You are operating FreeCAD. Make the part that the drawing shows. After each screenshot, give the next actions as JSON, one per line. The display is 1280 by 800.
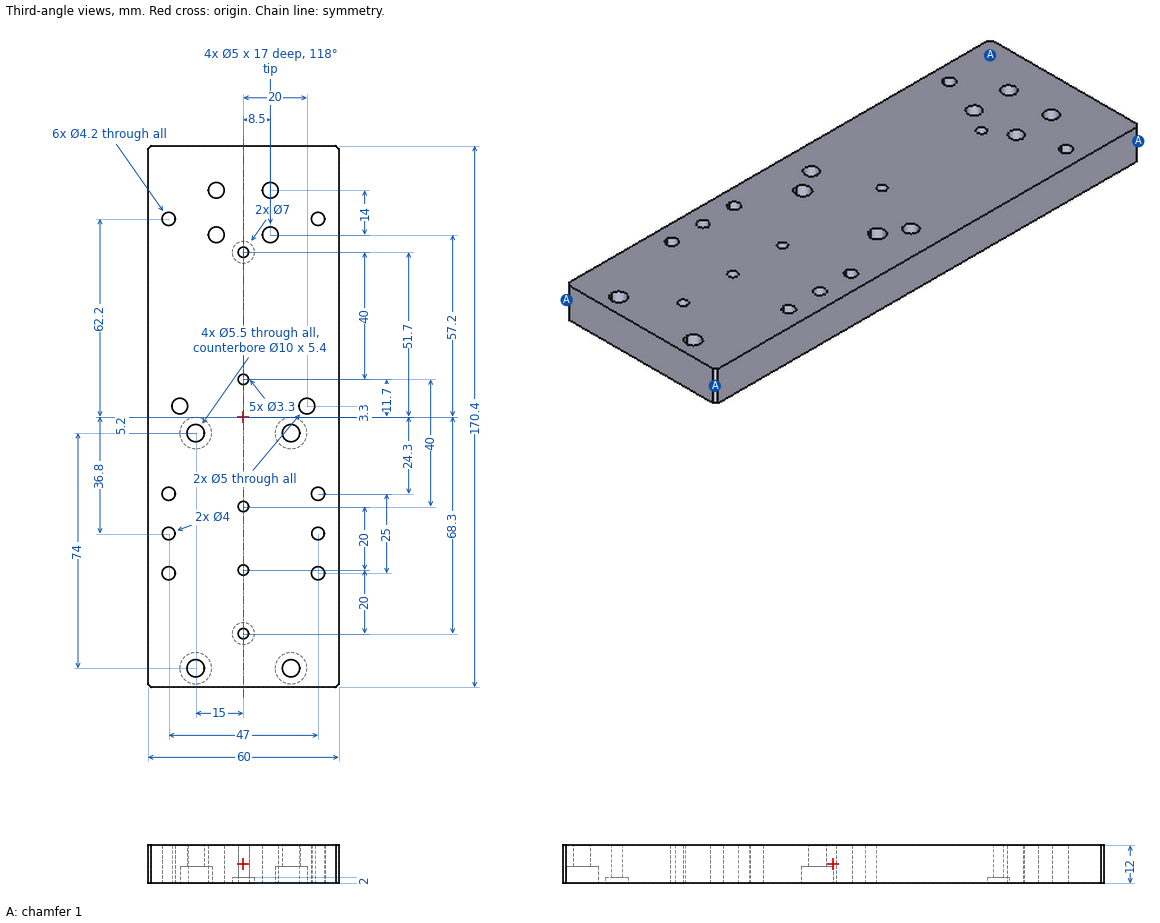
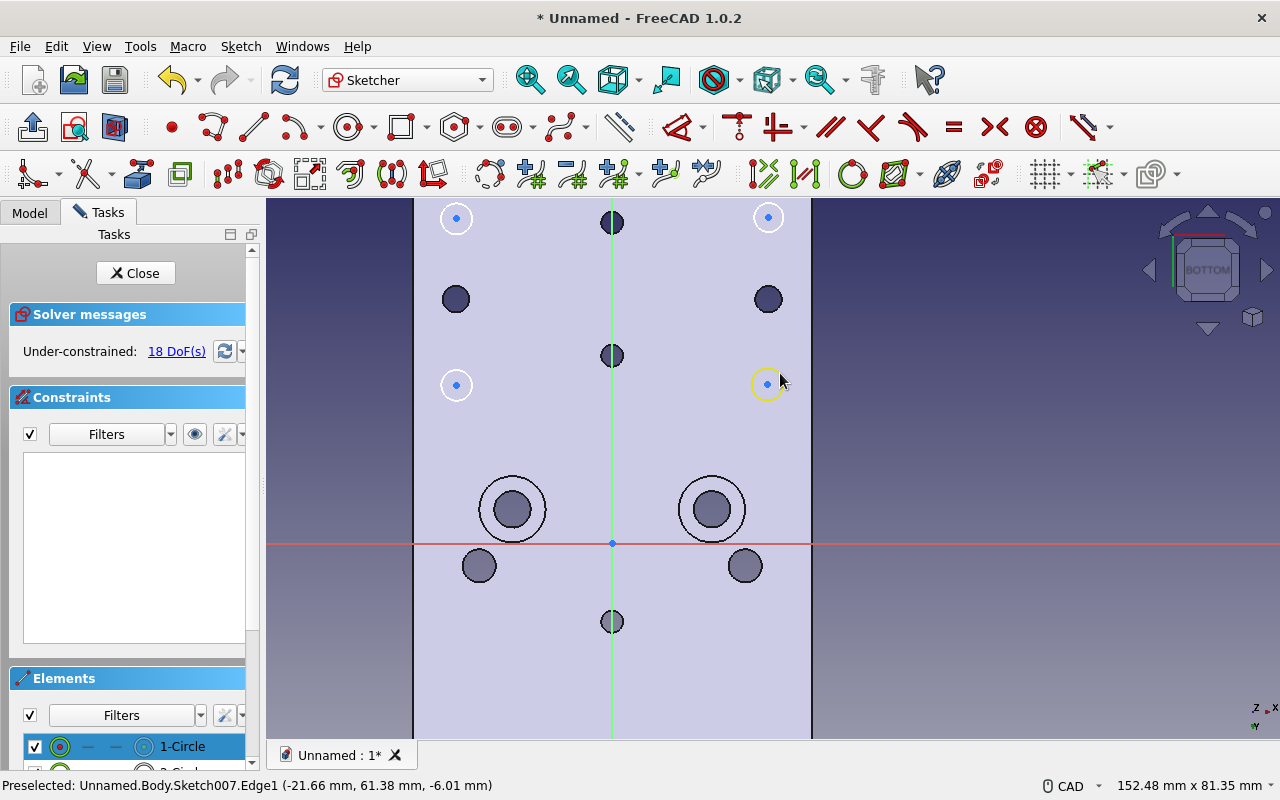
{"action": "left_click", "coordinate": [779, 373]}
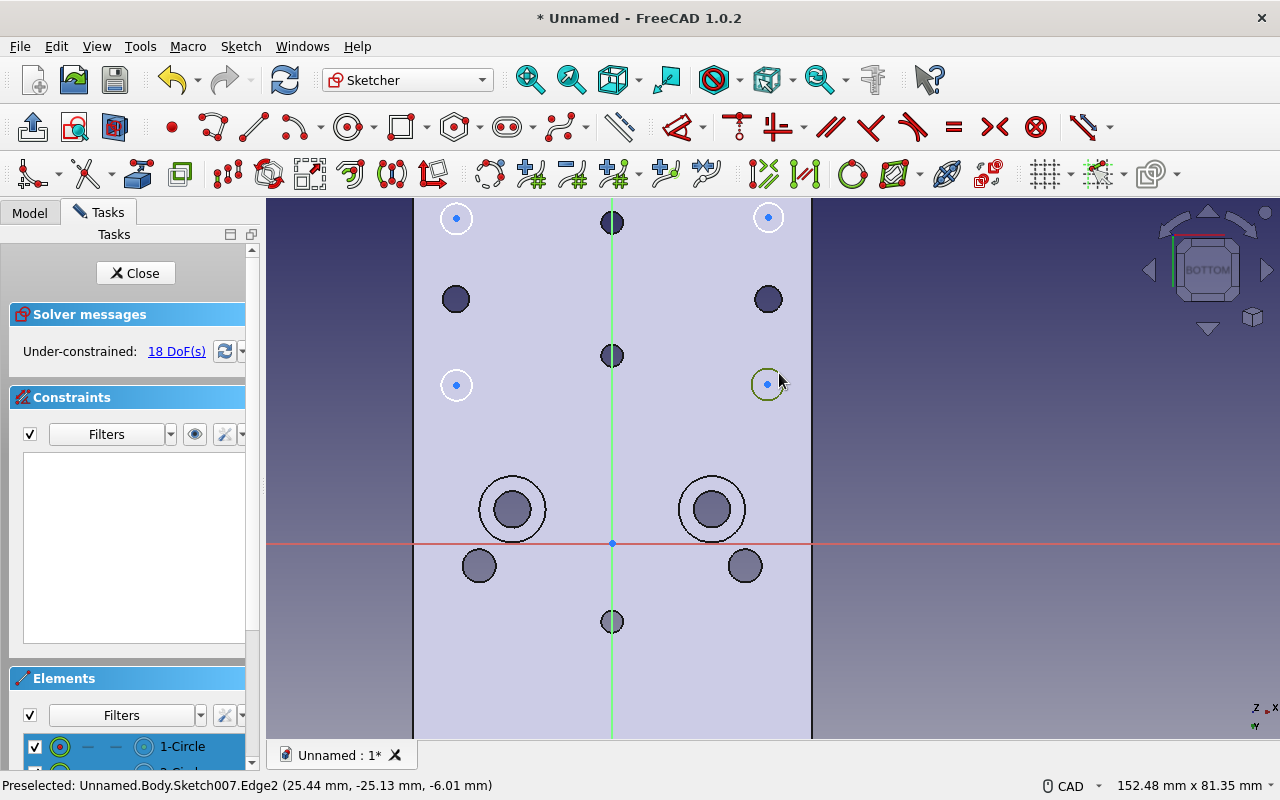
{"action": "left_click", "coordinate": [759, 228]}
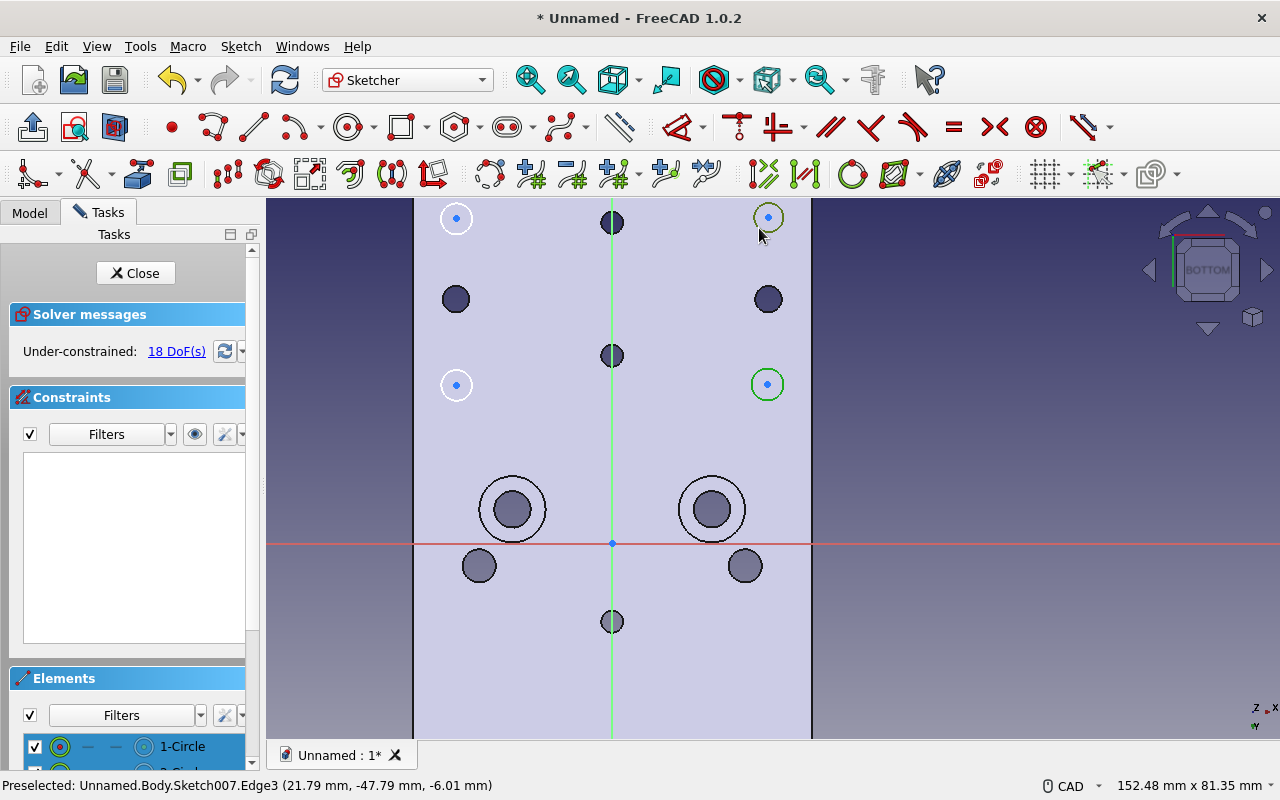
{"action": "left_click", "coordinate": [446, 230]}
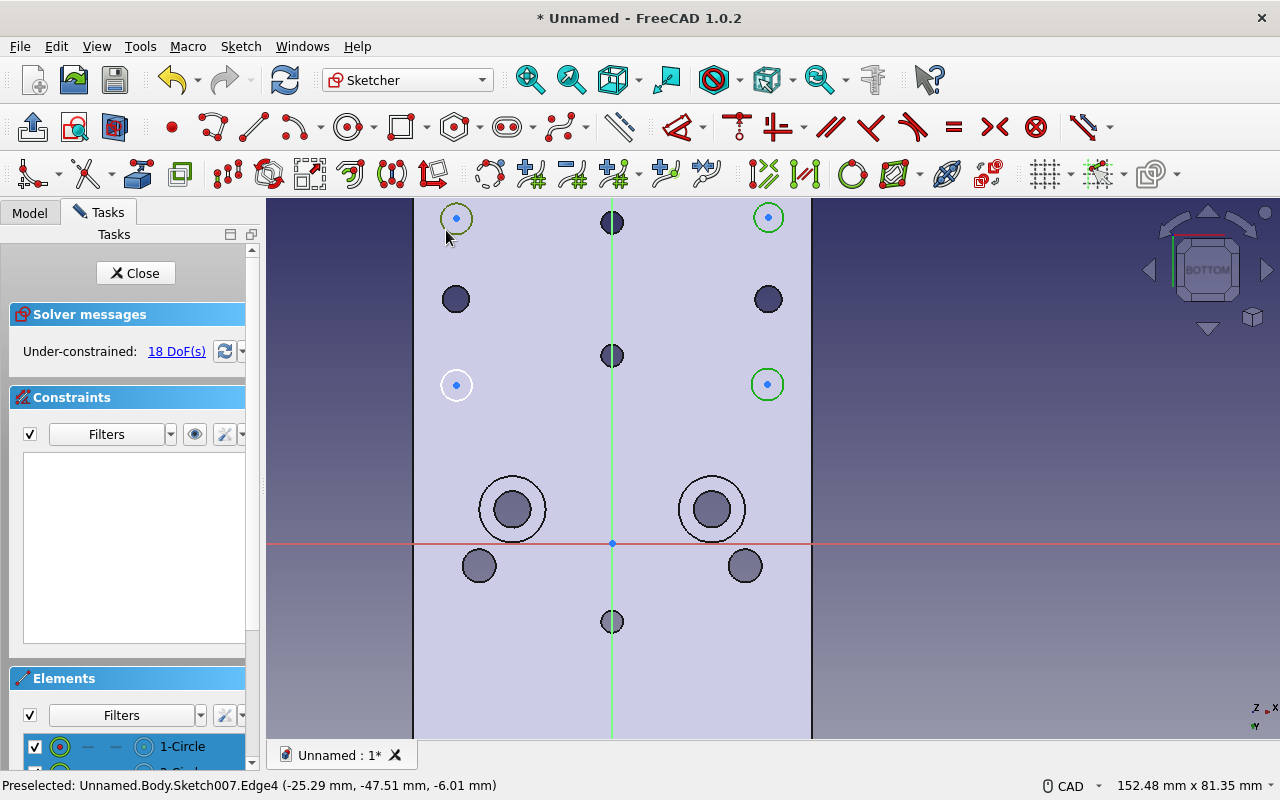
{"action": "left_click", "coordinate": [467, 375]}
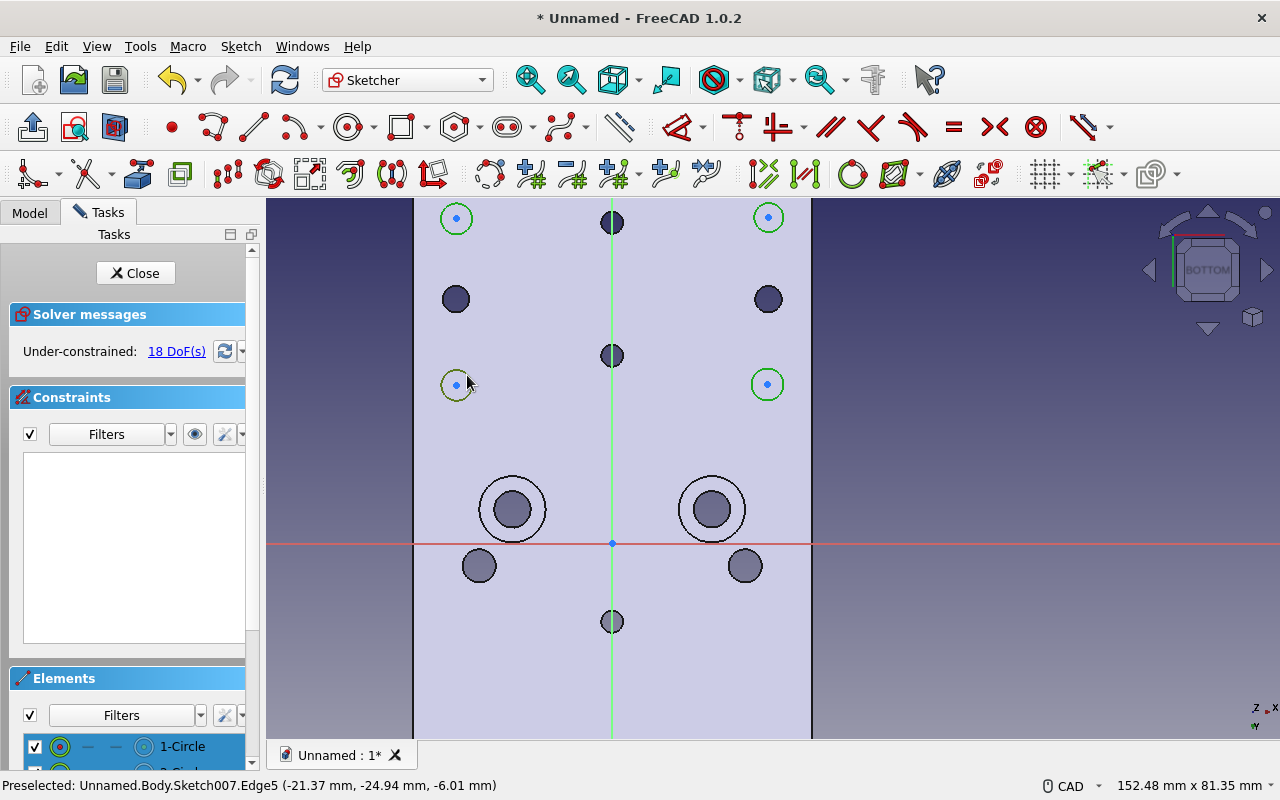
{"action": "scroll", "coordinate": [780, 372], "scroll_direction": "down", "scroll_amount": 4}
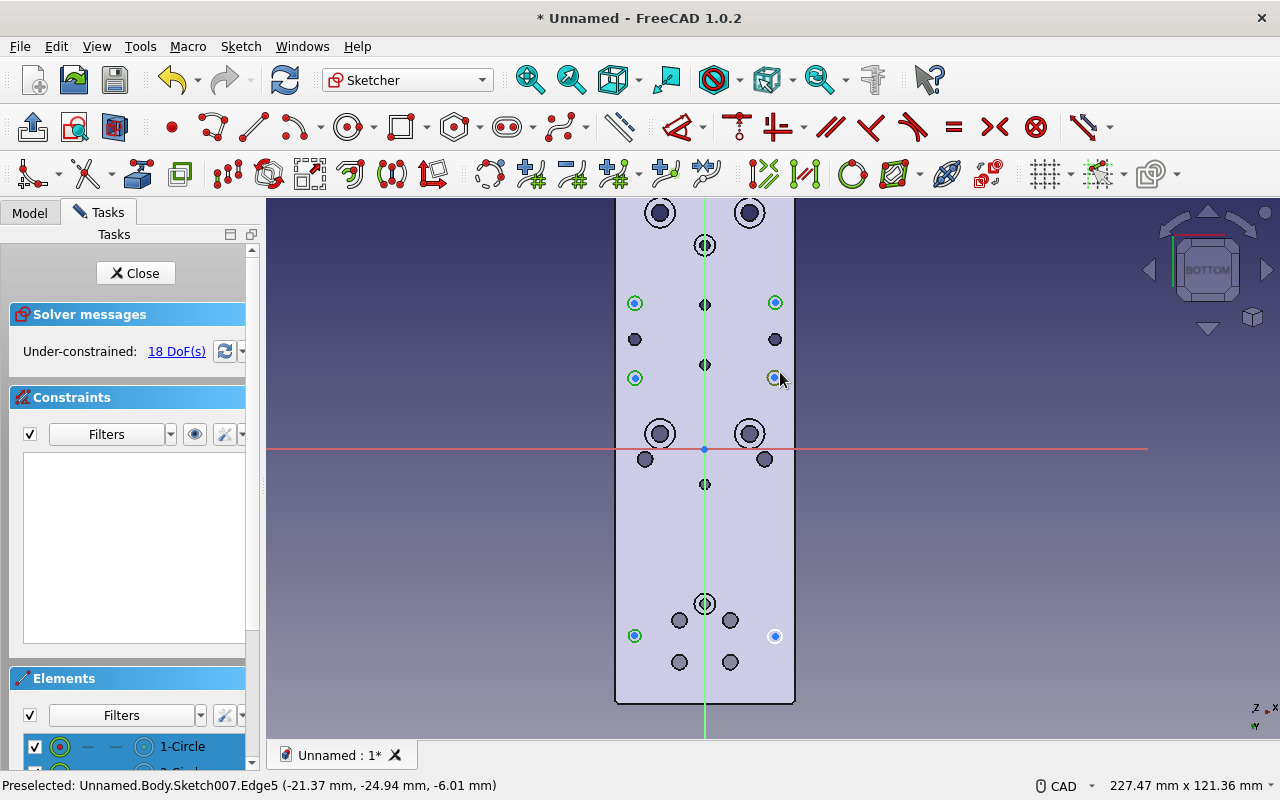
{"action": "scroll", "coordinate": [780, 632], "scroll_direction": "up", "scroll_amount": 4}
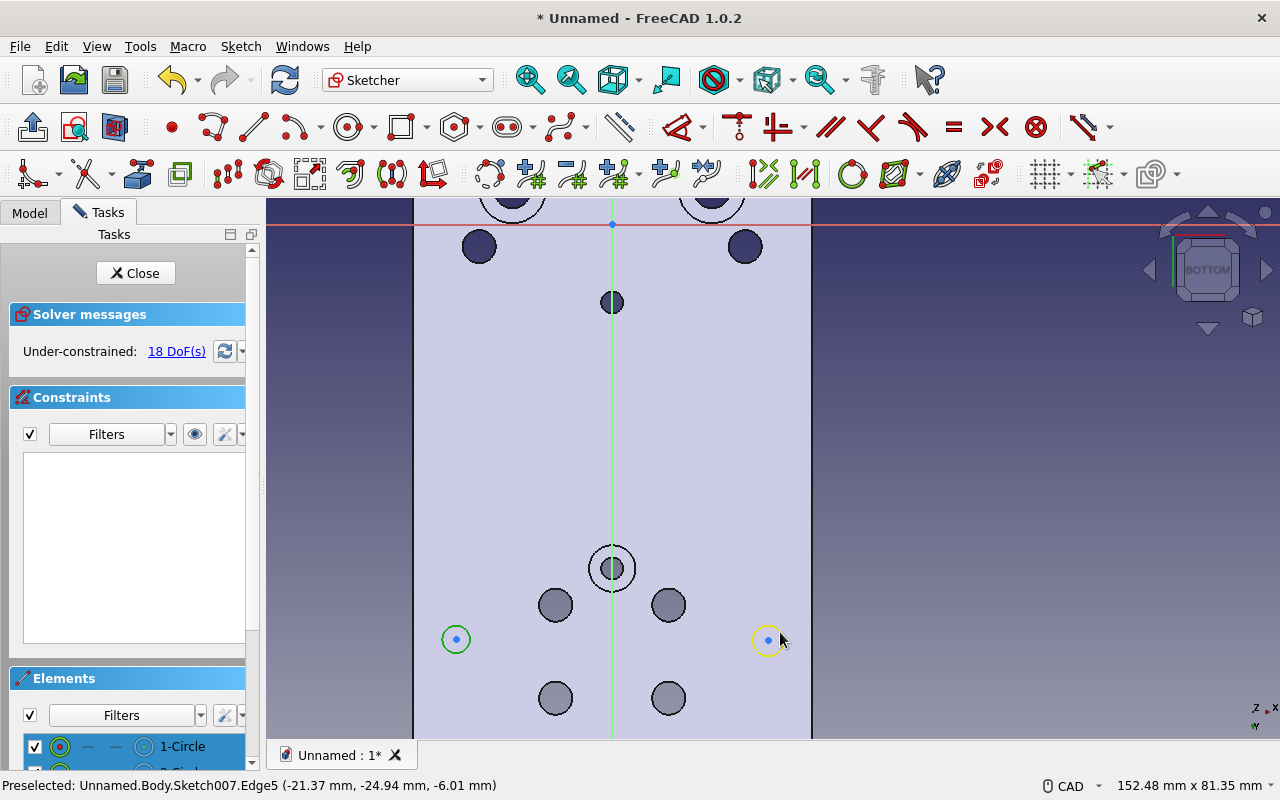
{"action": "left_click", "coordinate": [779, 630]}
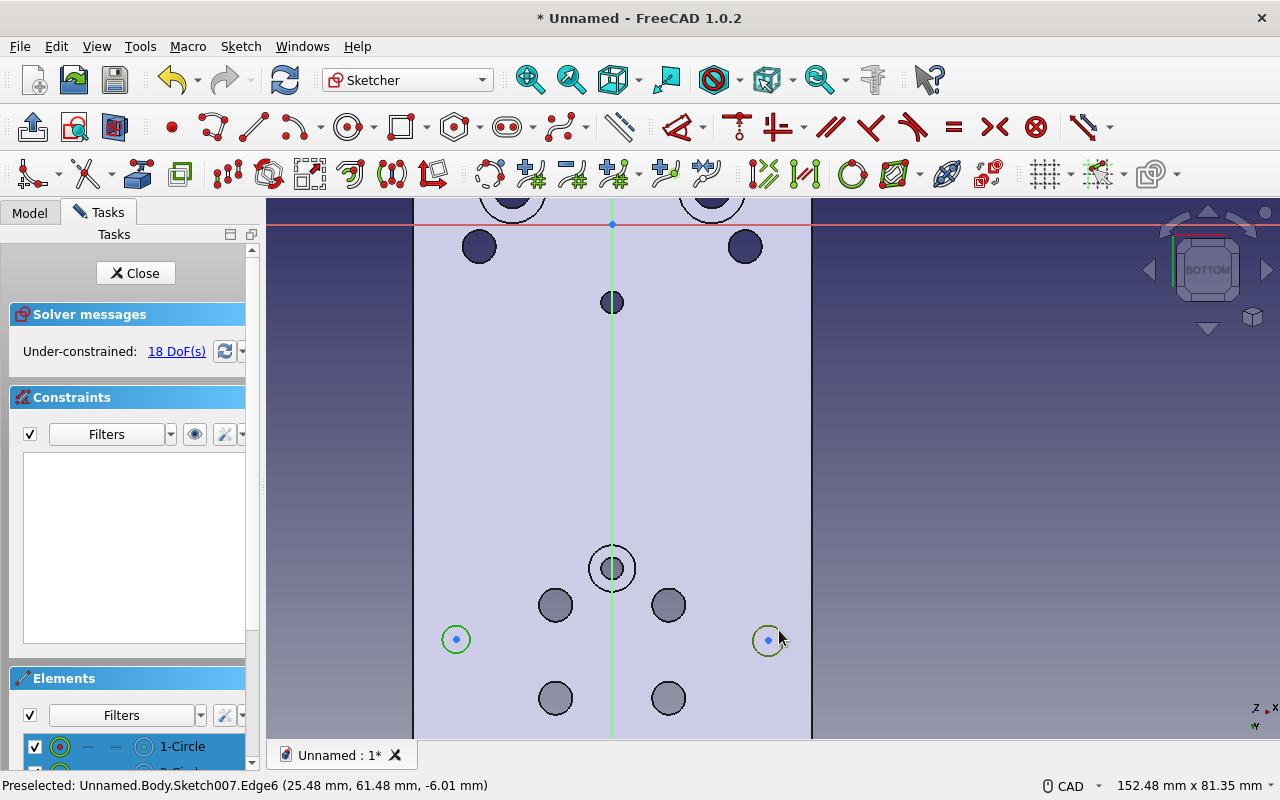
{"action": "left_click", "coordinate": [954, 128]}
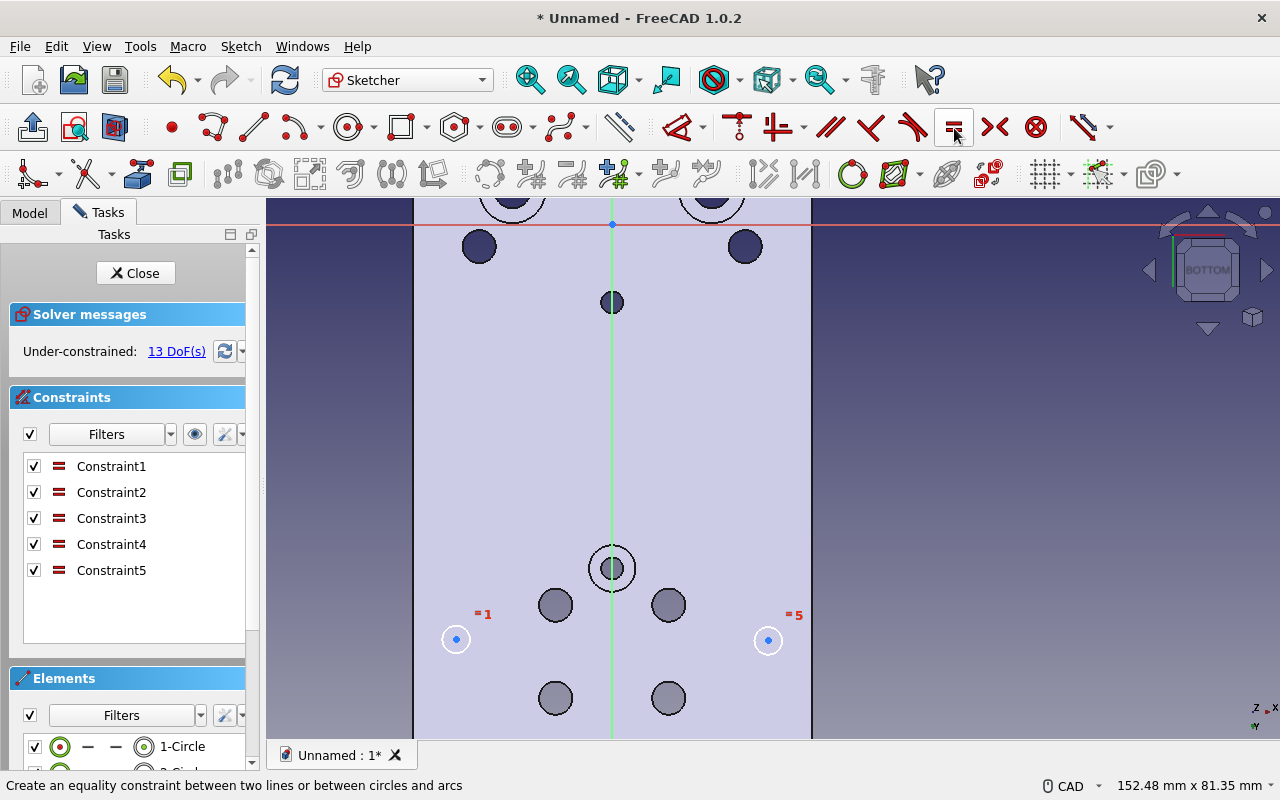
{"action": "scroll", "coordinate": [780, 632], "scroll_direction": "down", "scroll_amount": 4}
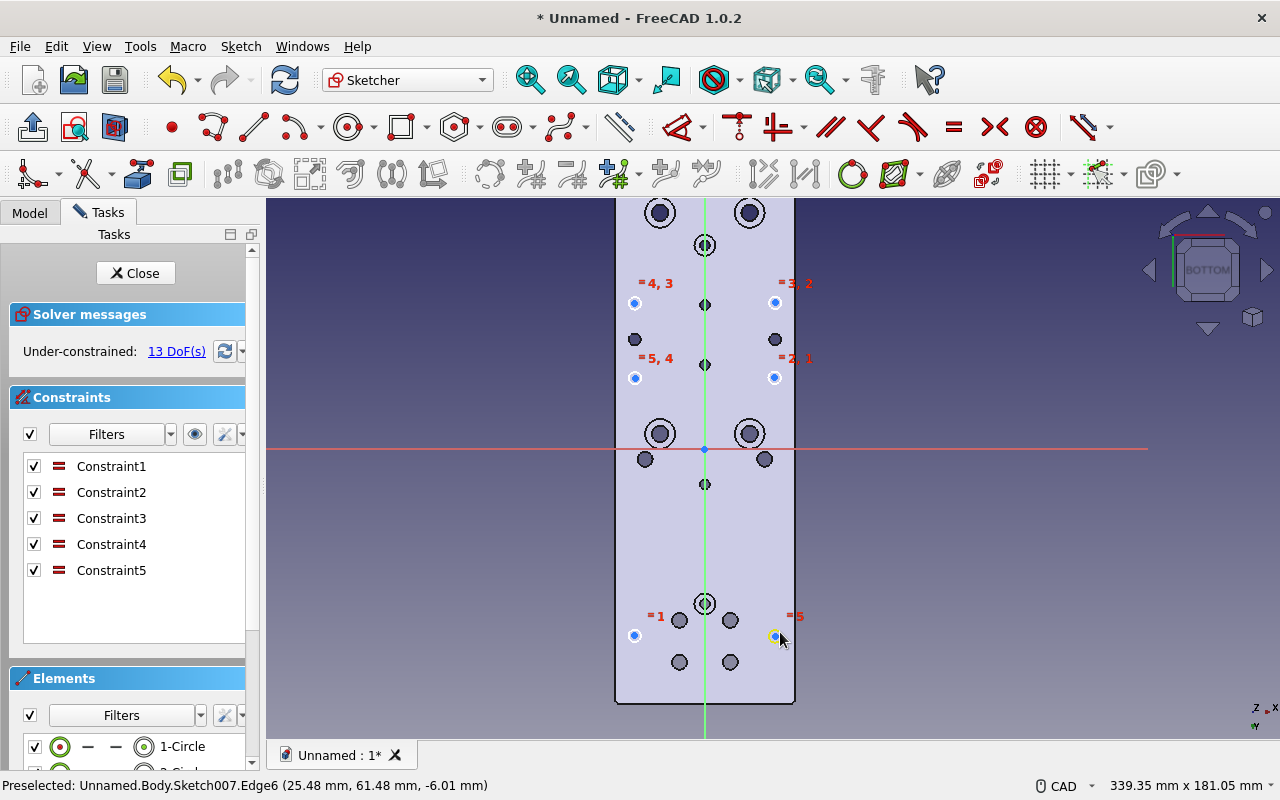
{"action": "left_click", "coordinate": [775, 303]}